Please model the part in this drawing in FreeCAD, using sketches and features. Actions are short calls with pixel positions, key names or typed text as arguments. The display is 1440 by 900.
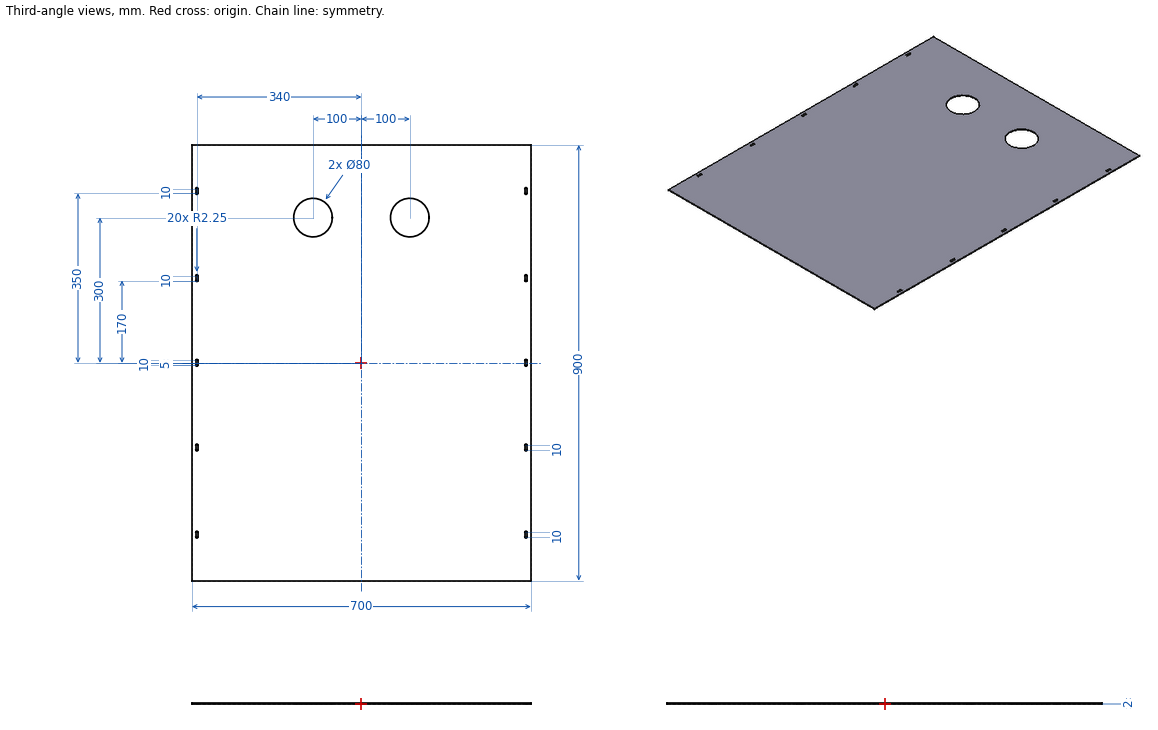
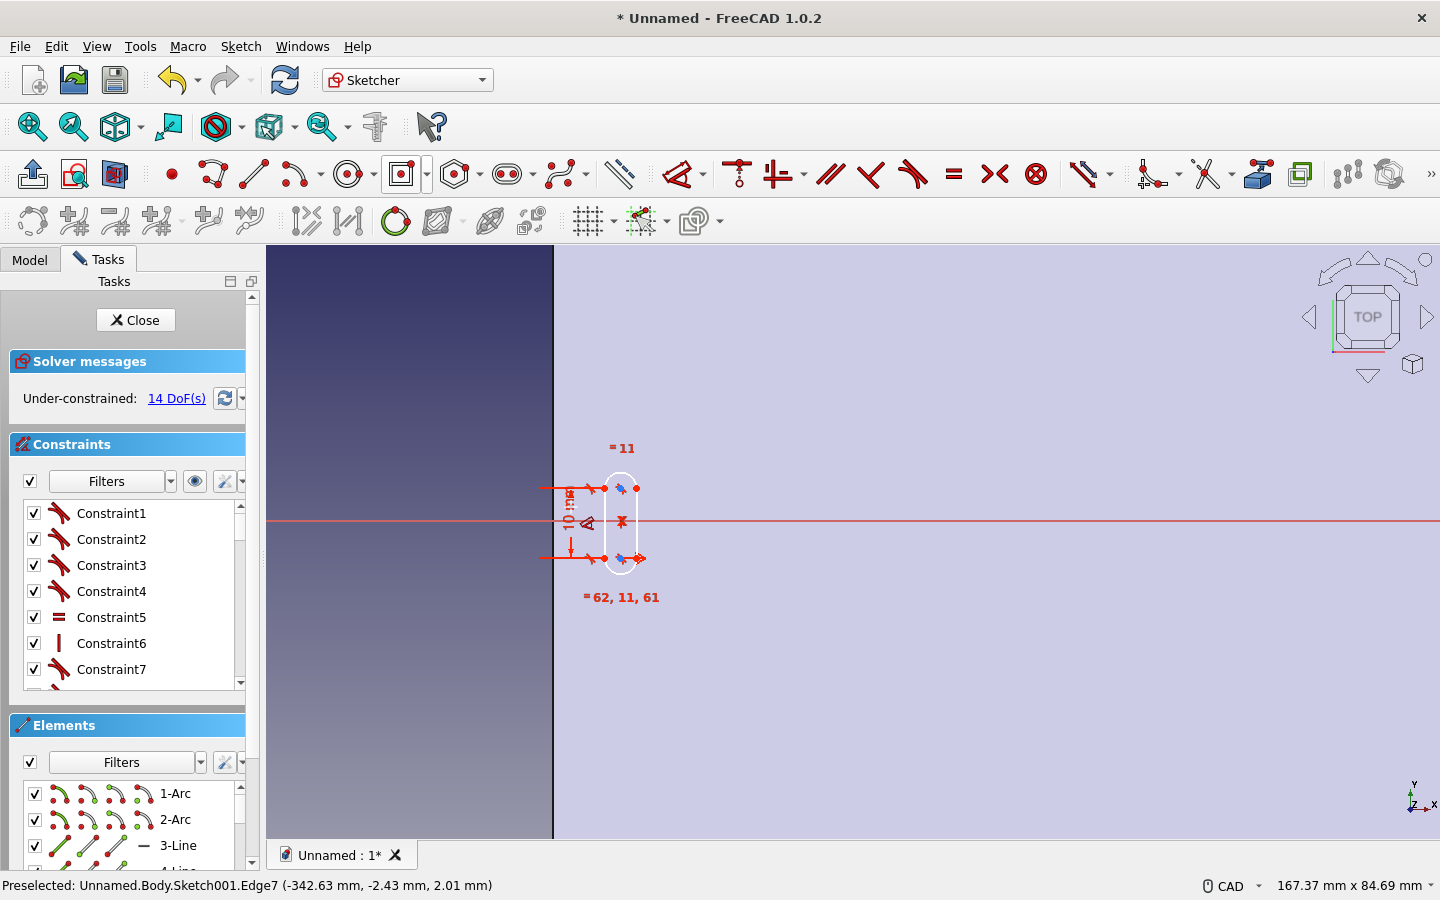
scroll(606, 544, down, 13)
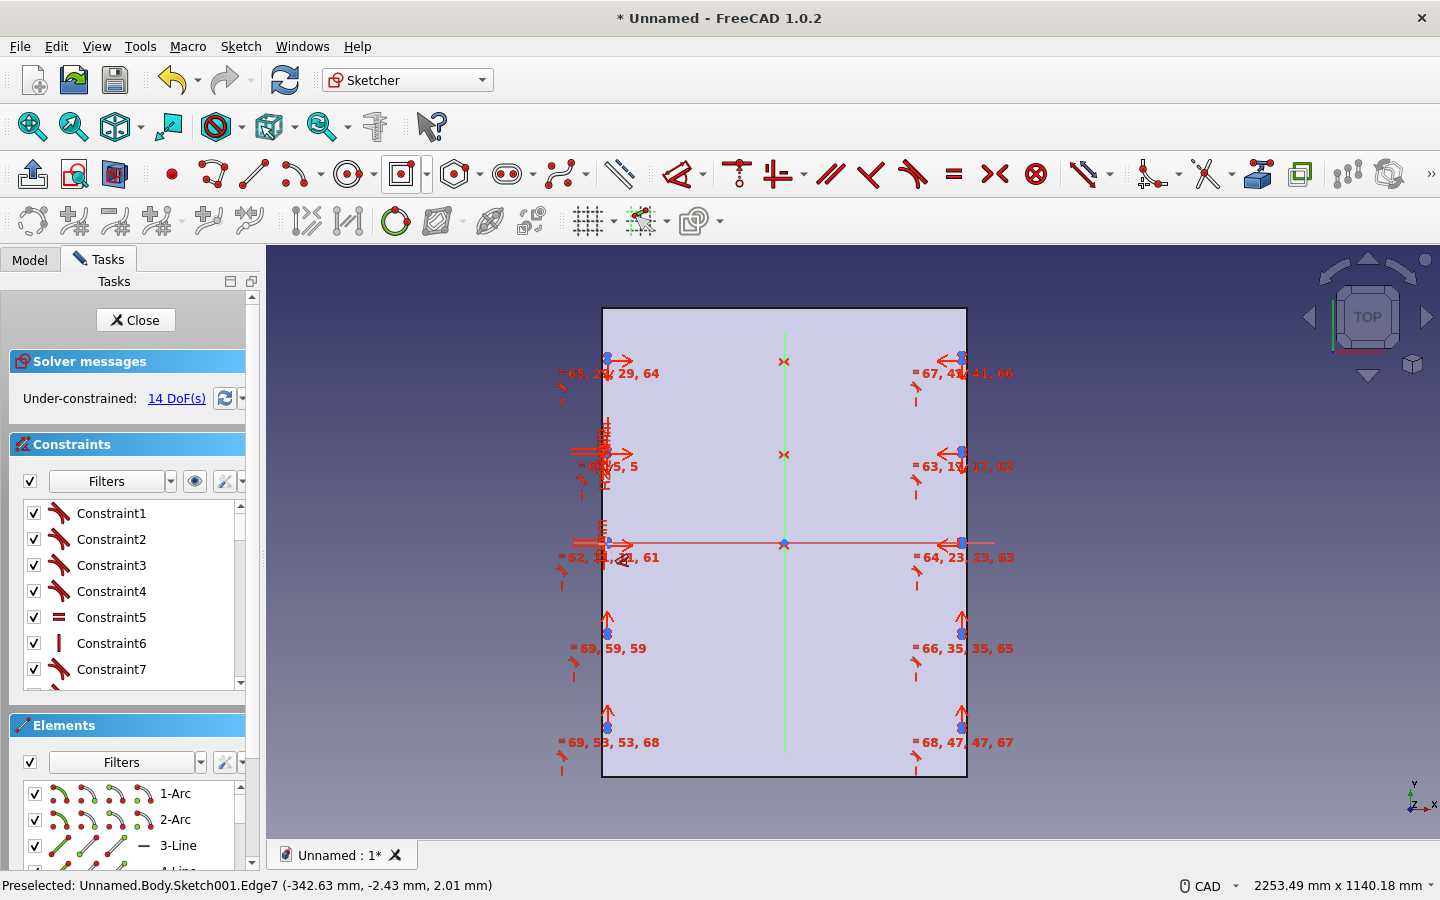
scroll(961, 453, up, 12)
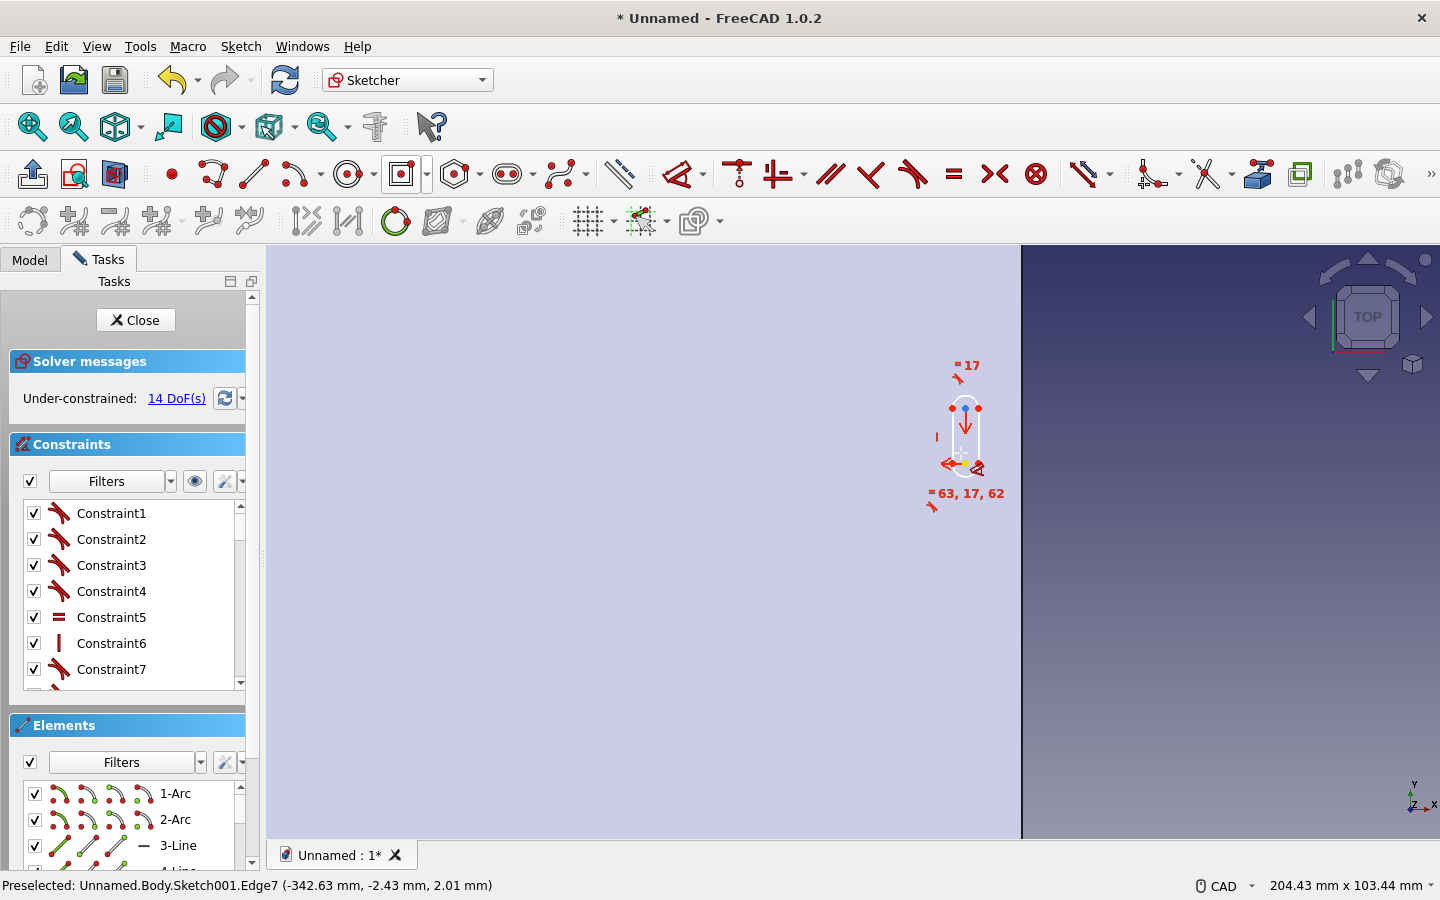
click(953, 447)
click(919, 436)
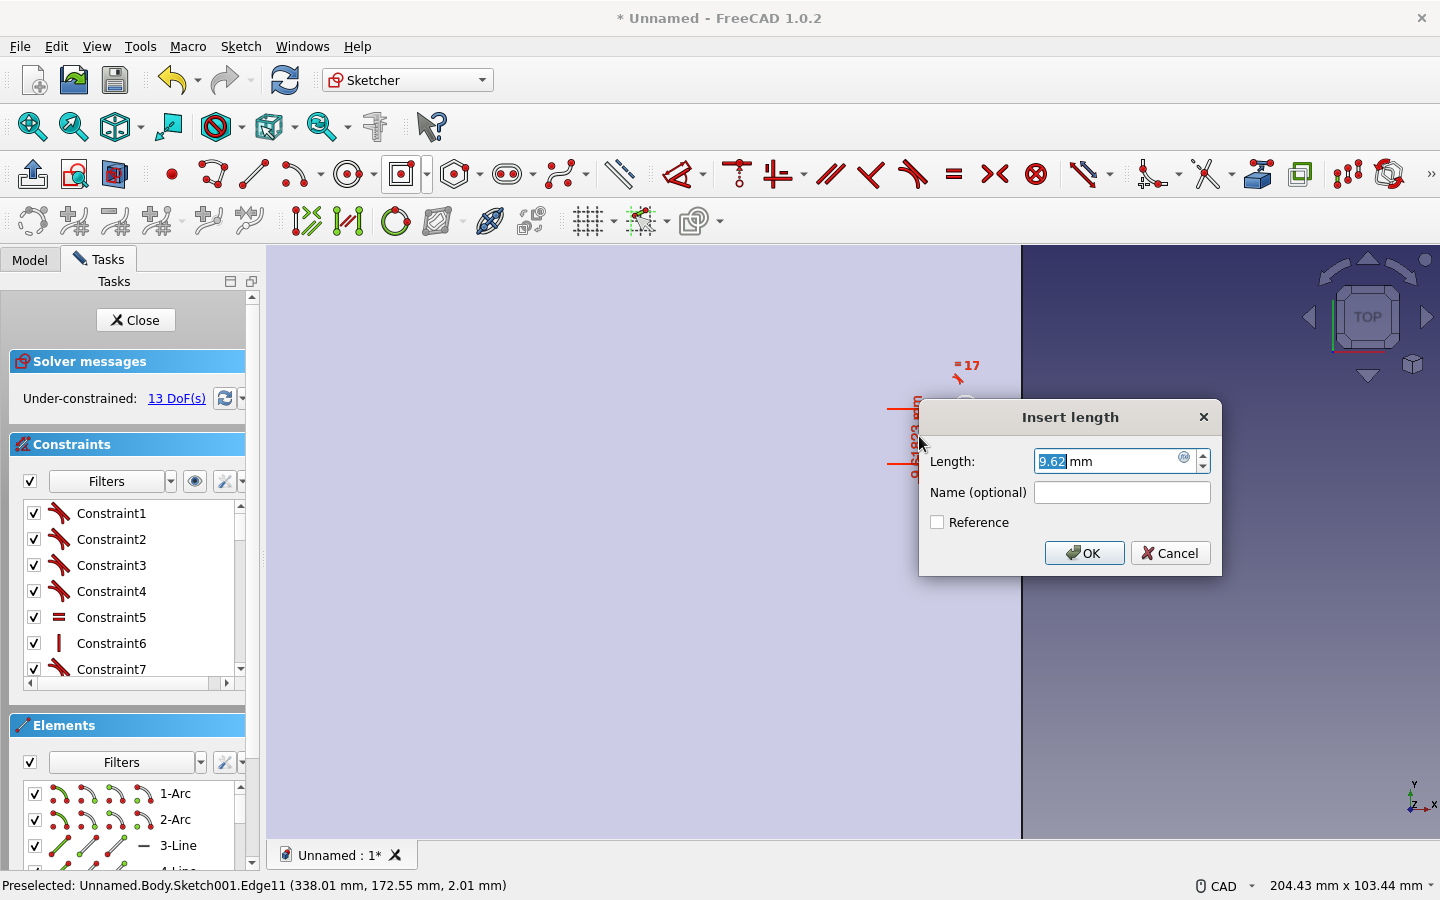
text(10)
key(Return)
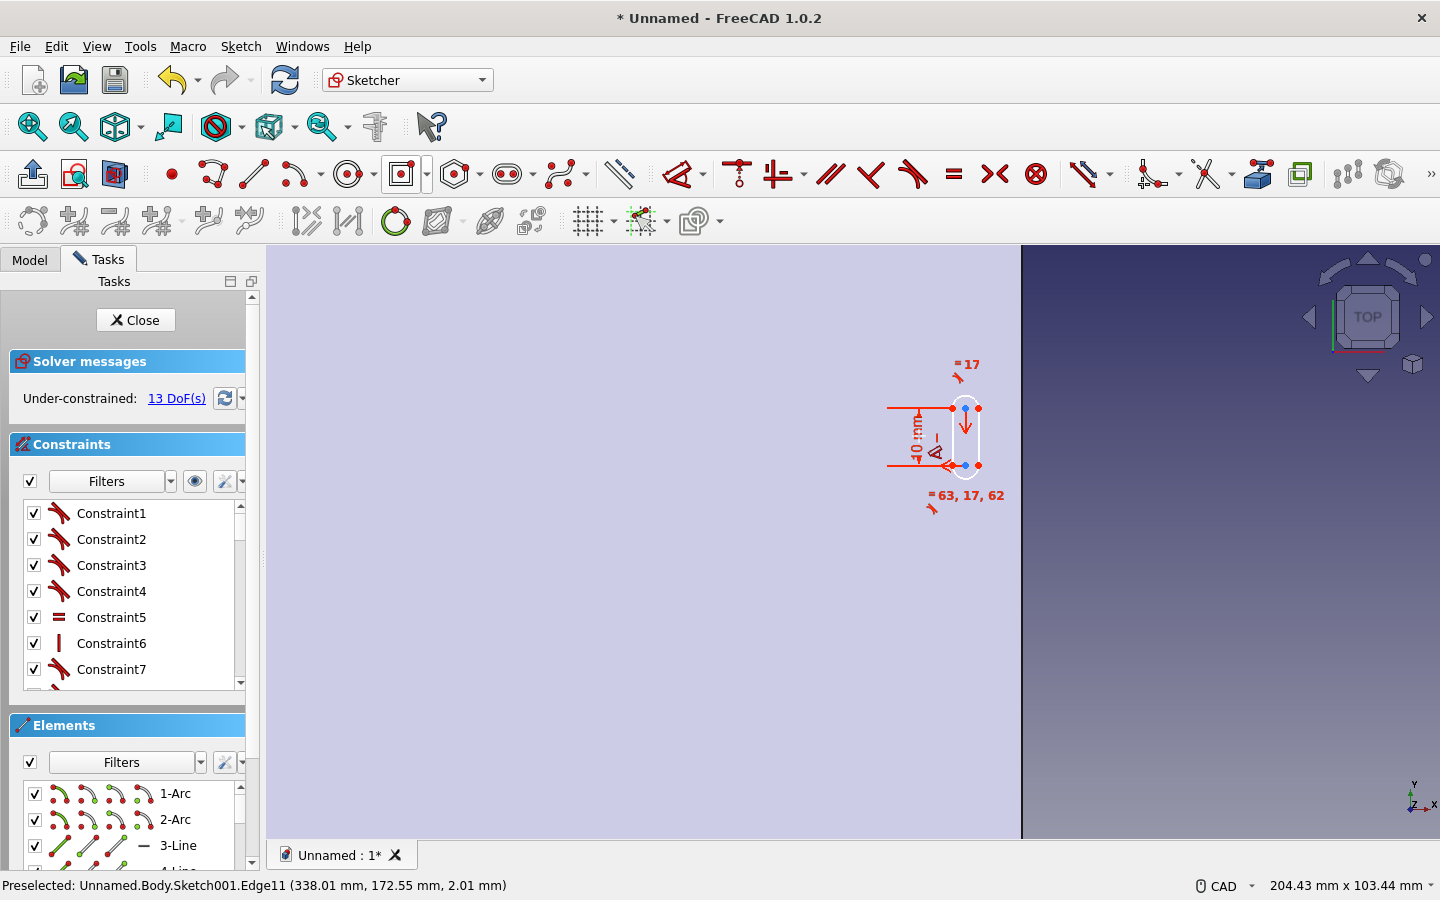
scroll(961, 453, down, 12)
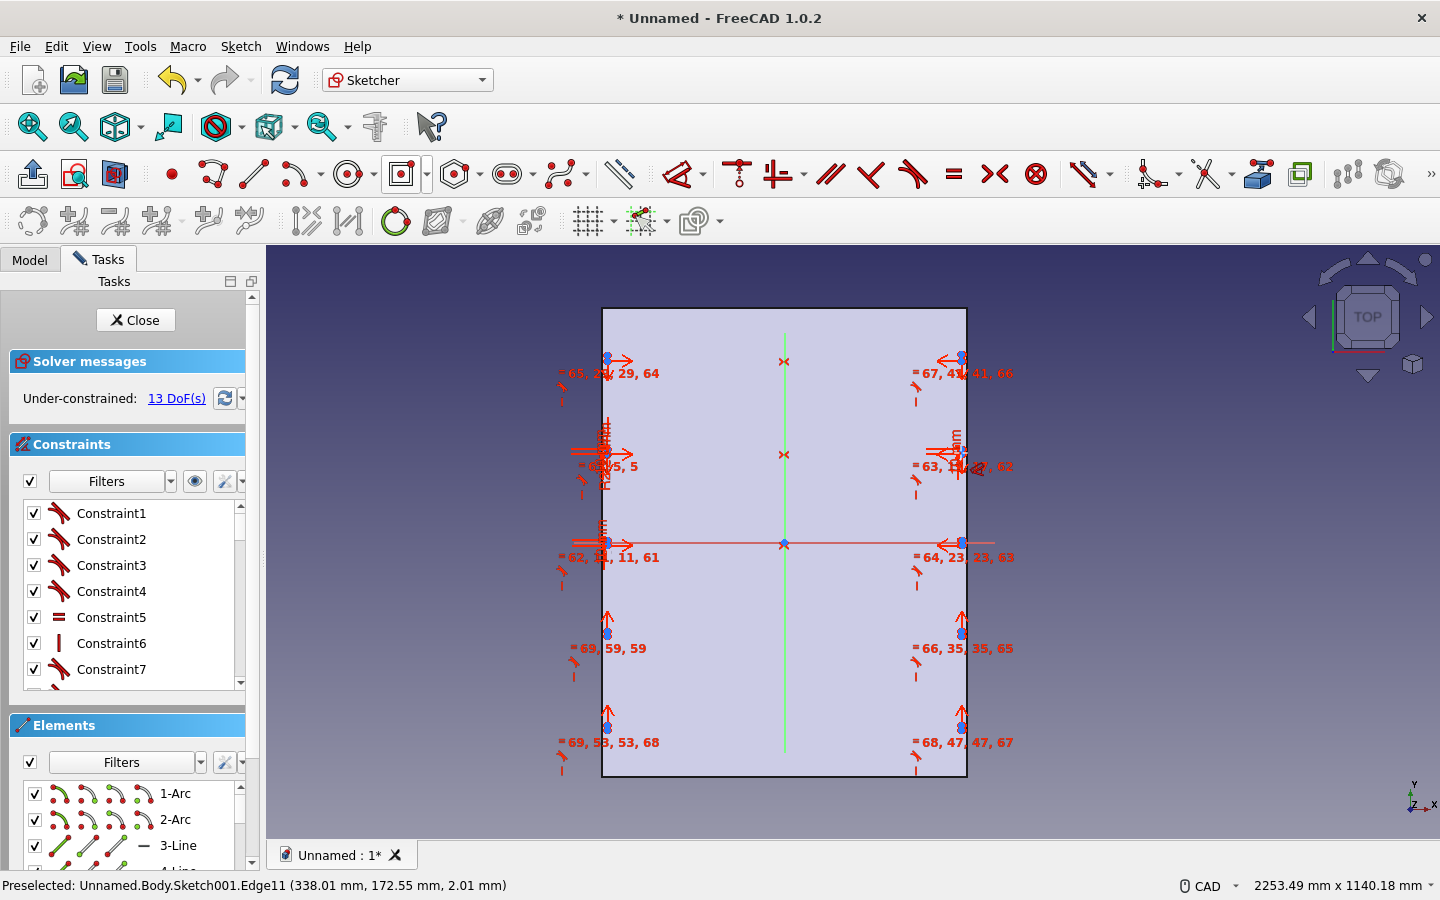
scroll(961, 544, up, 13)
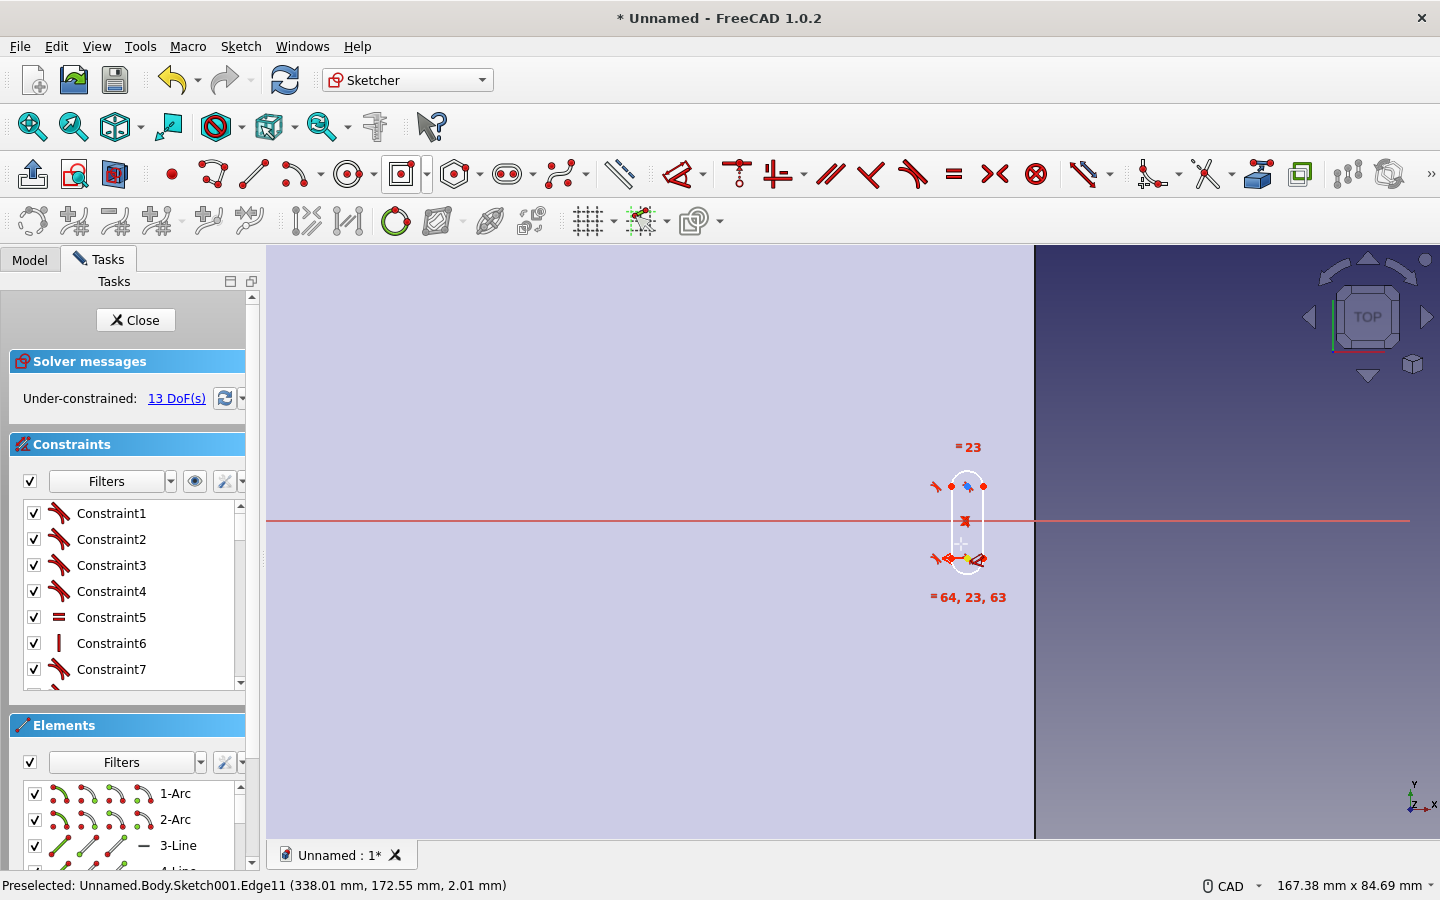
click(952, 537)
click(918, 506)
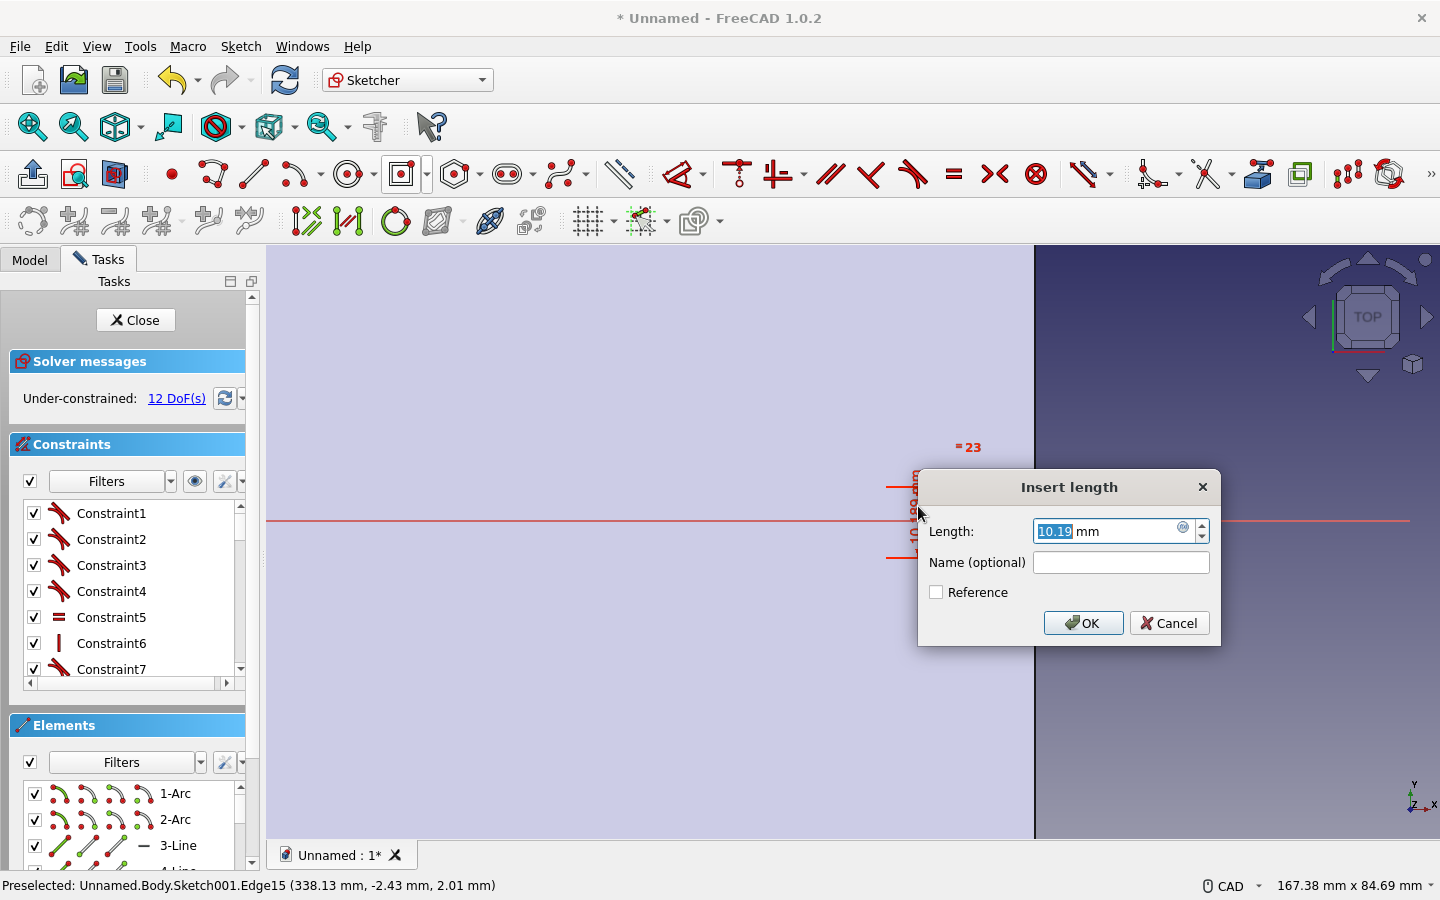
text(10)
key(Return)